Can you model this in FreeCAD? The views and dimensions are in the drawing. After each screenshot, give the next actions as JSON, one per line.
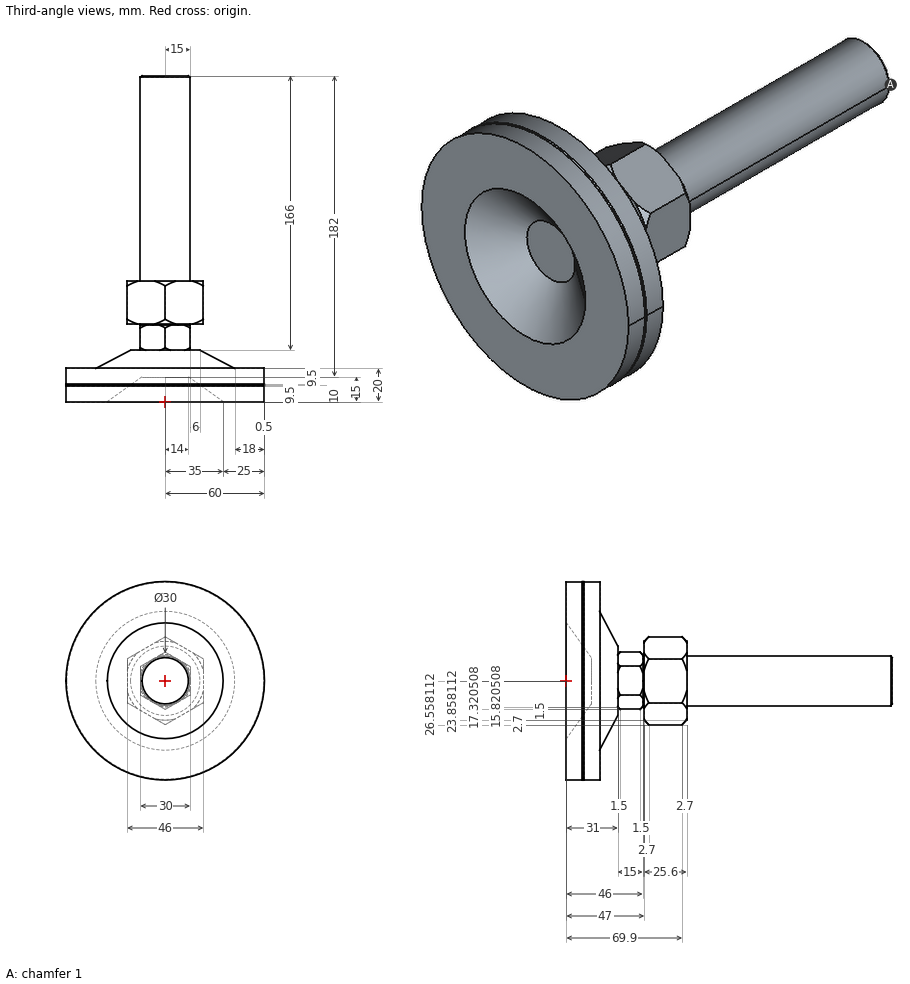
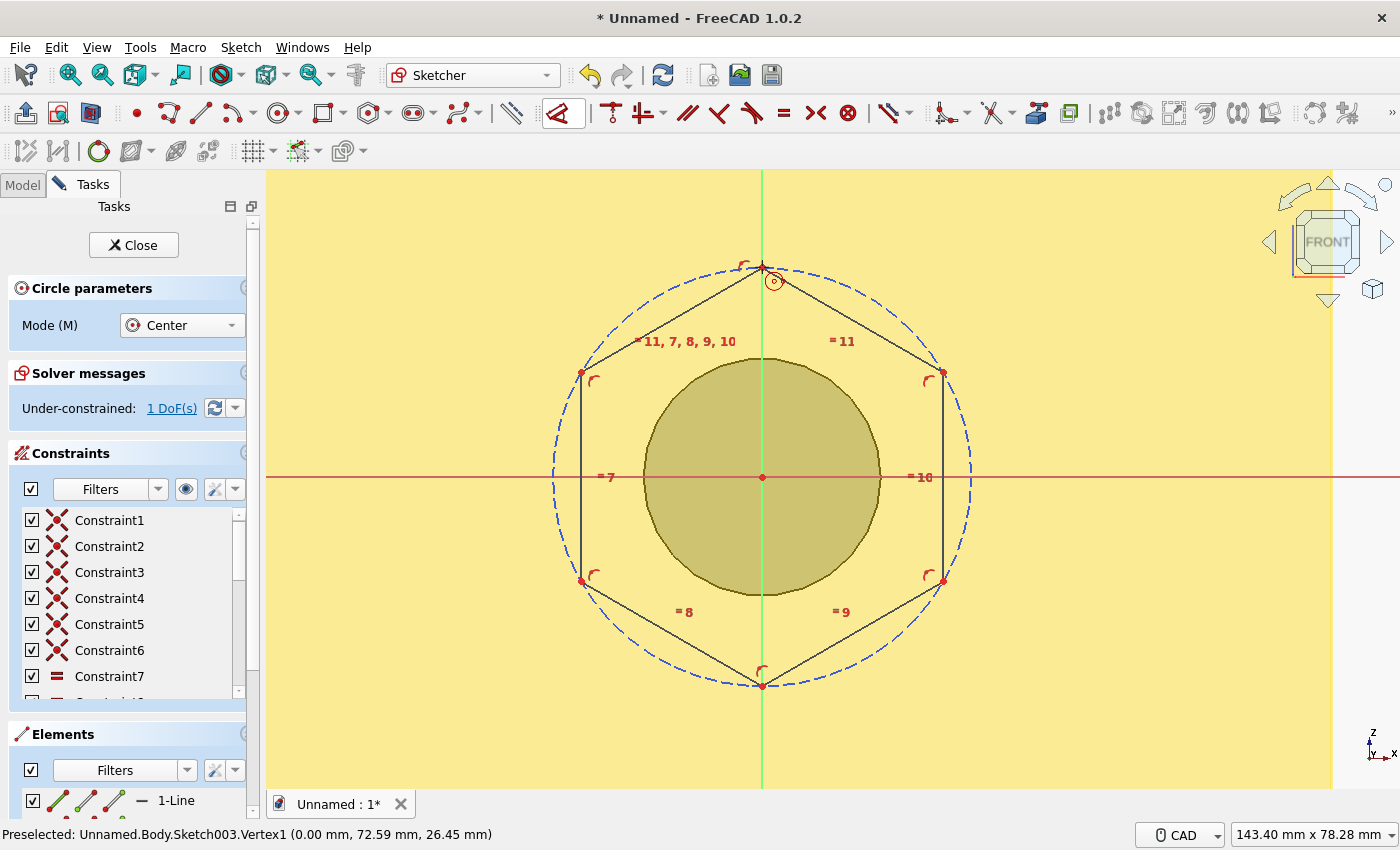
{"action": "left_click", "coordinate": [762, 477]}
{"action": "mouse_move", "coordinate": [846, 393]}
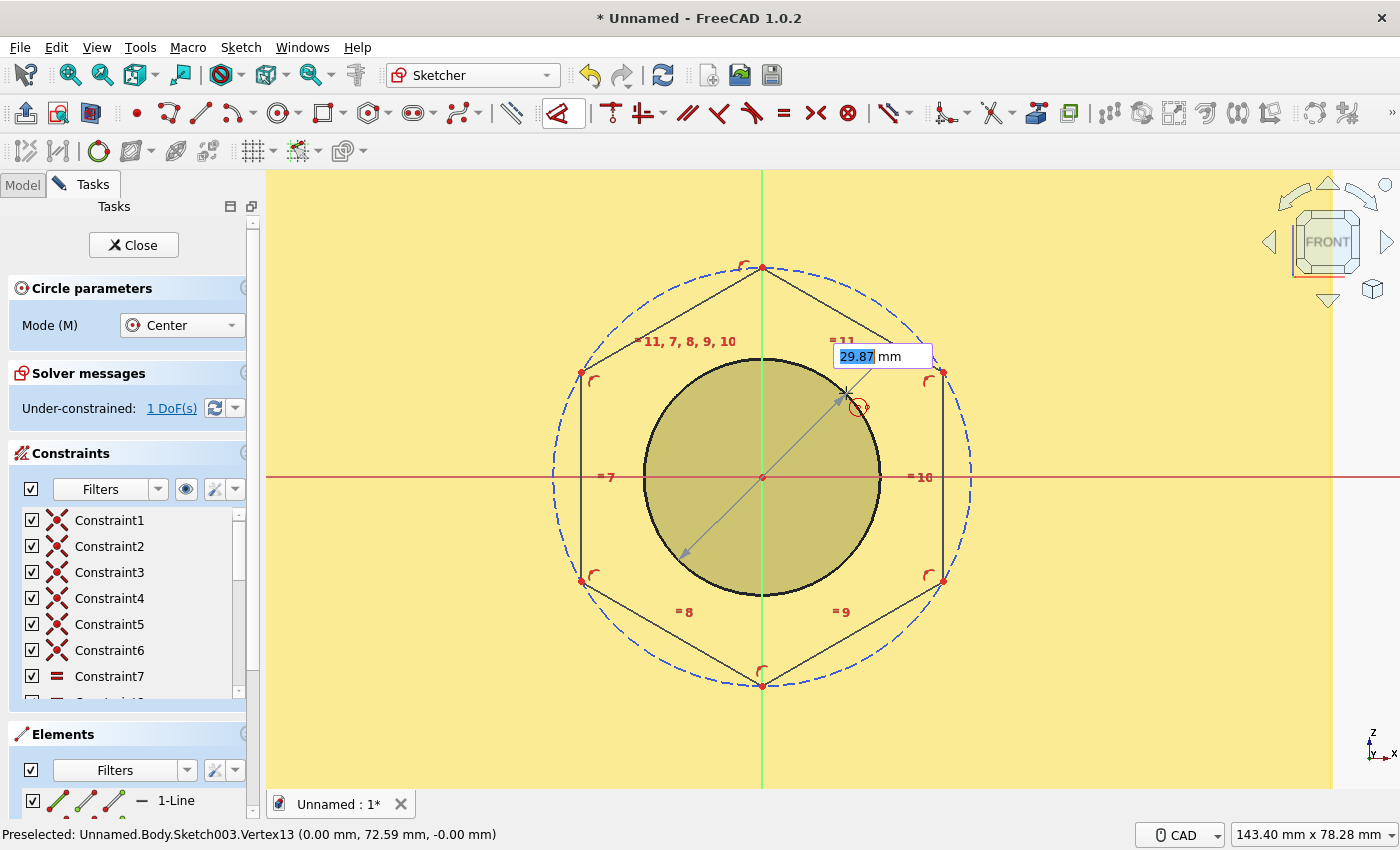
{"action": "type", "text": "30"}
{"action": "key", "text": "Return"}
{"action": "key", "text": "Escape"}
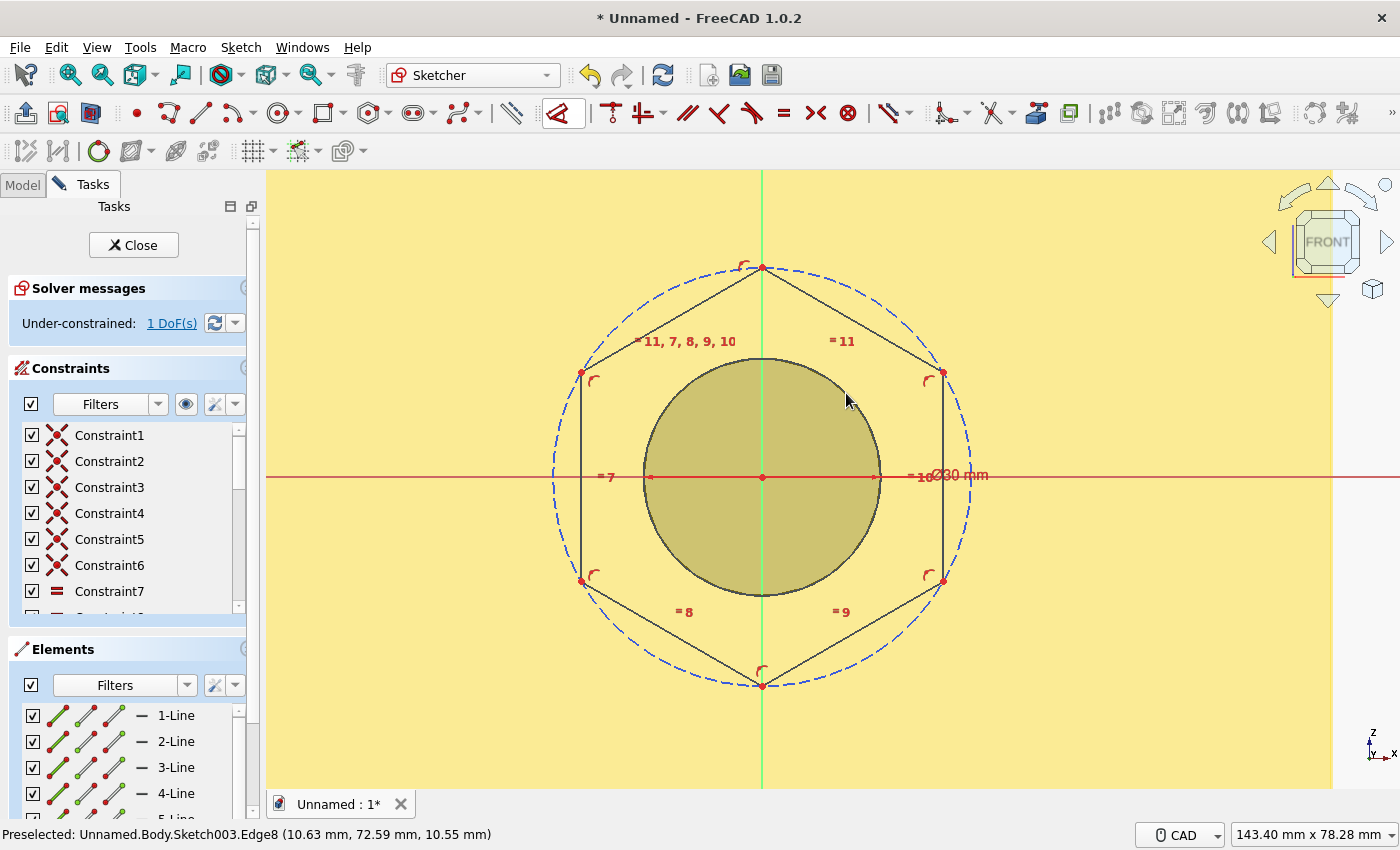
{"action": "left_click", "coordinate": [581, 373]}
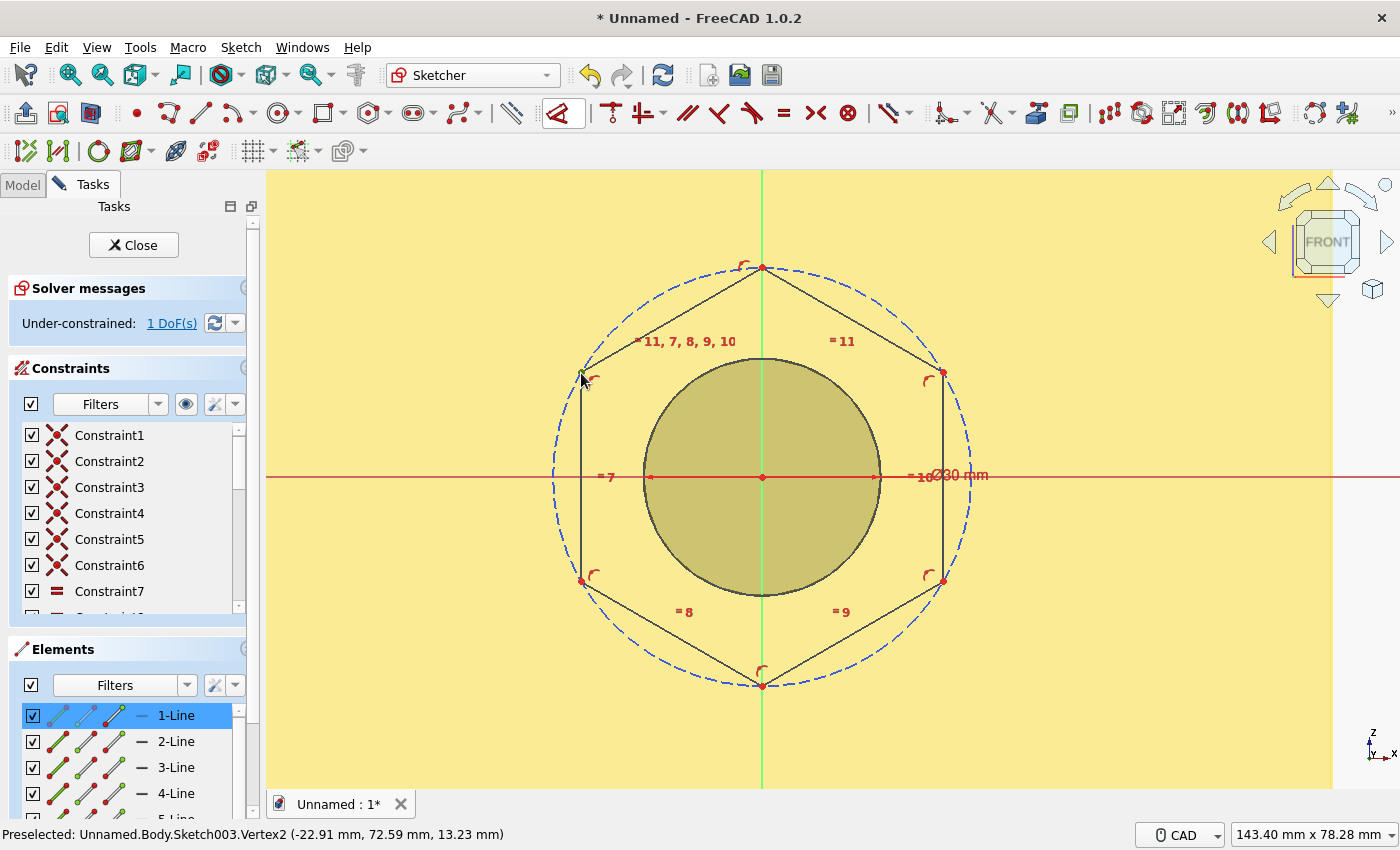
{"action": "left_click", "coordinate": [943, 582]}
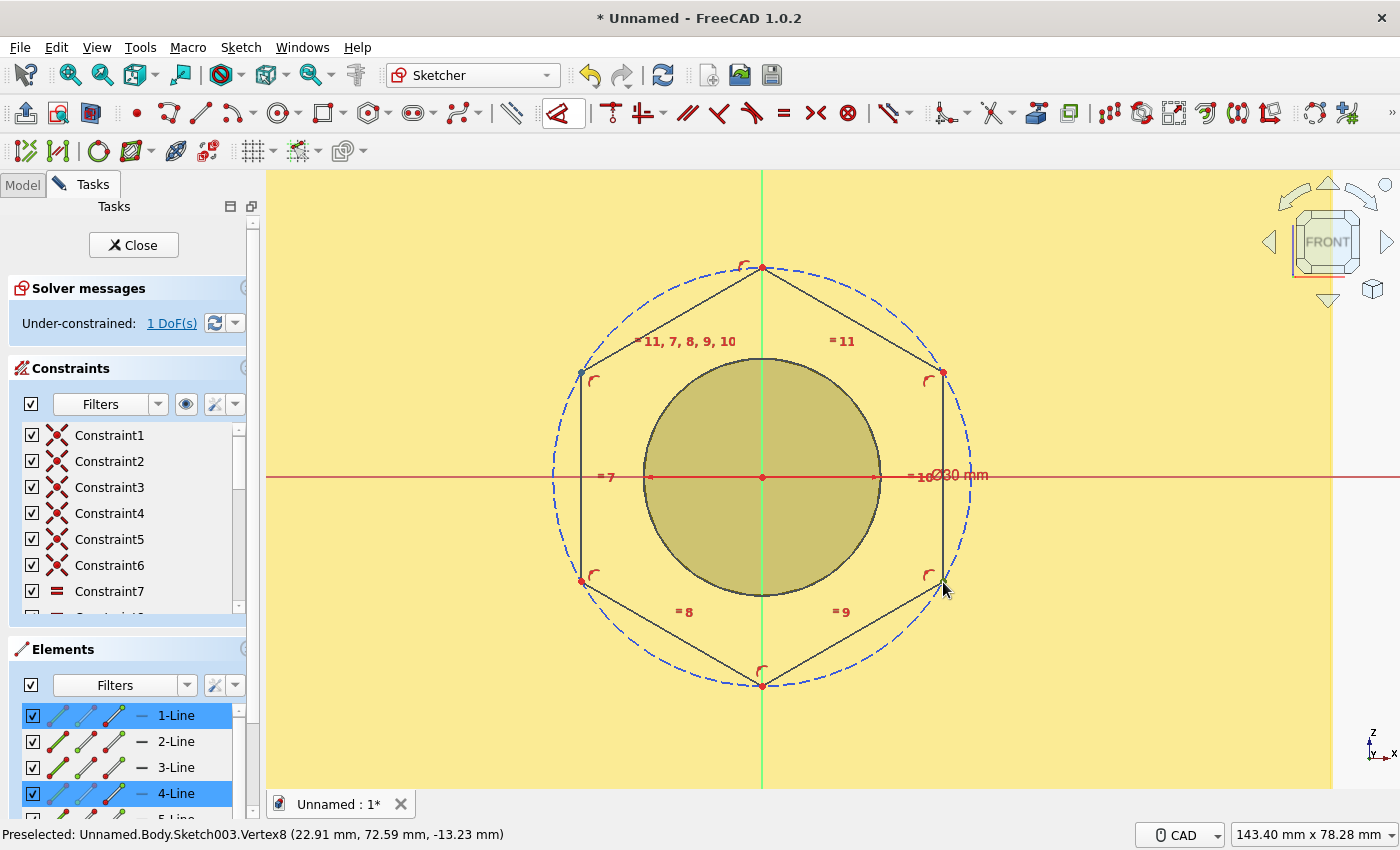
{"action": "key", "text": "l"}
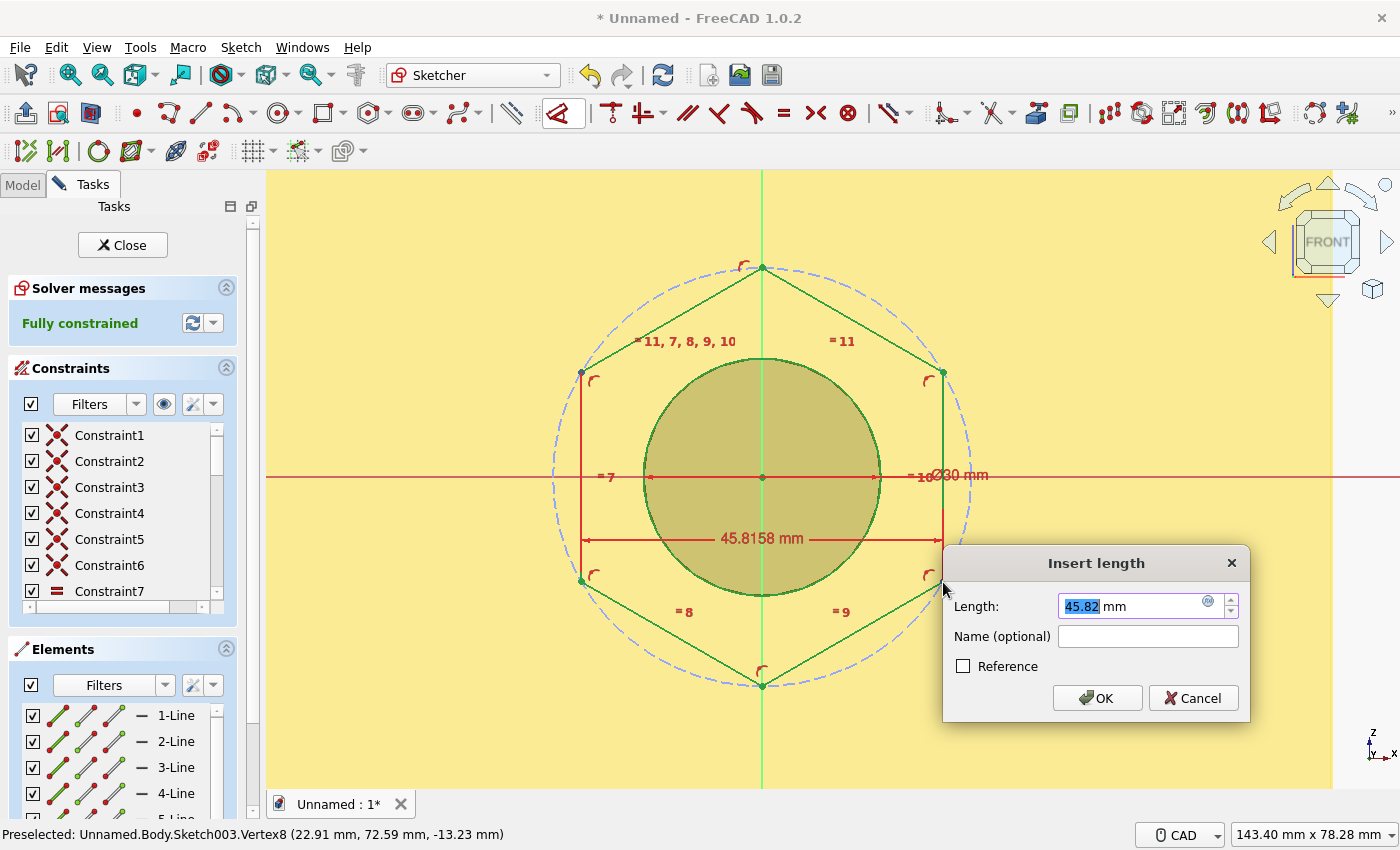
{"action": "type", "text": "46"}
{"action": "key", "text": "Return"}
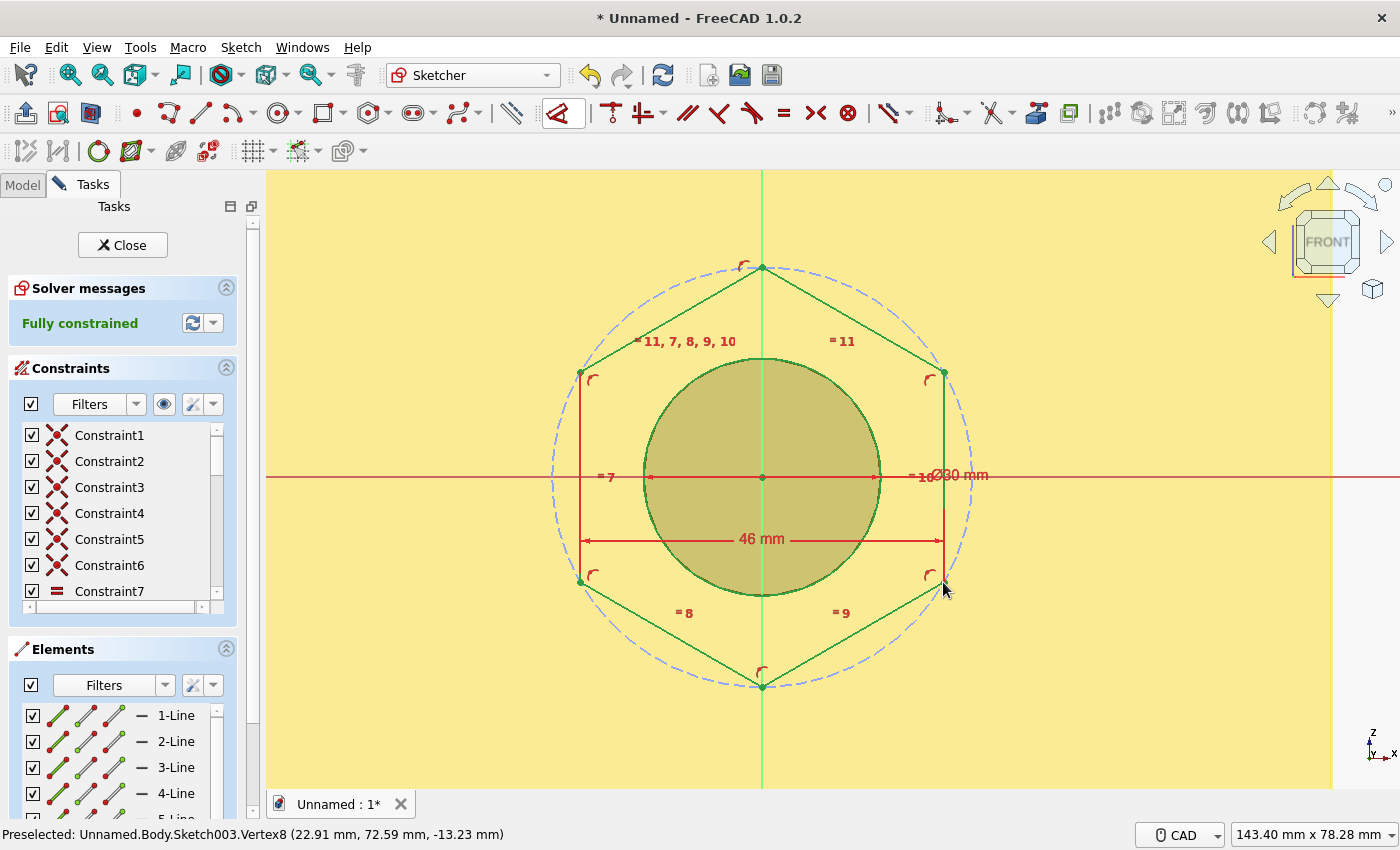
{"action": "left_click", "coordinate": [123, 245]}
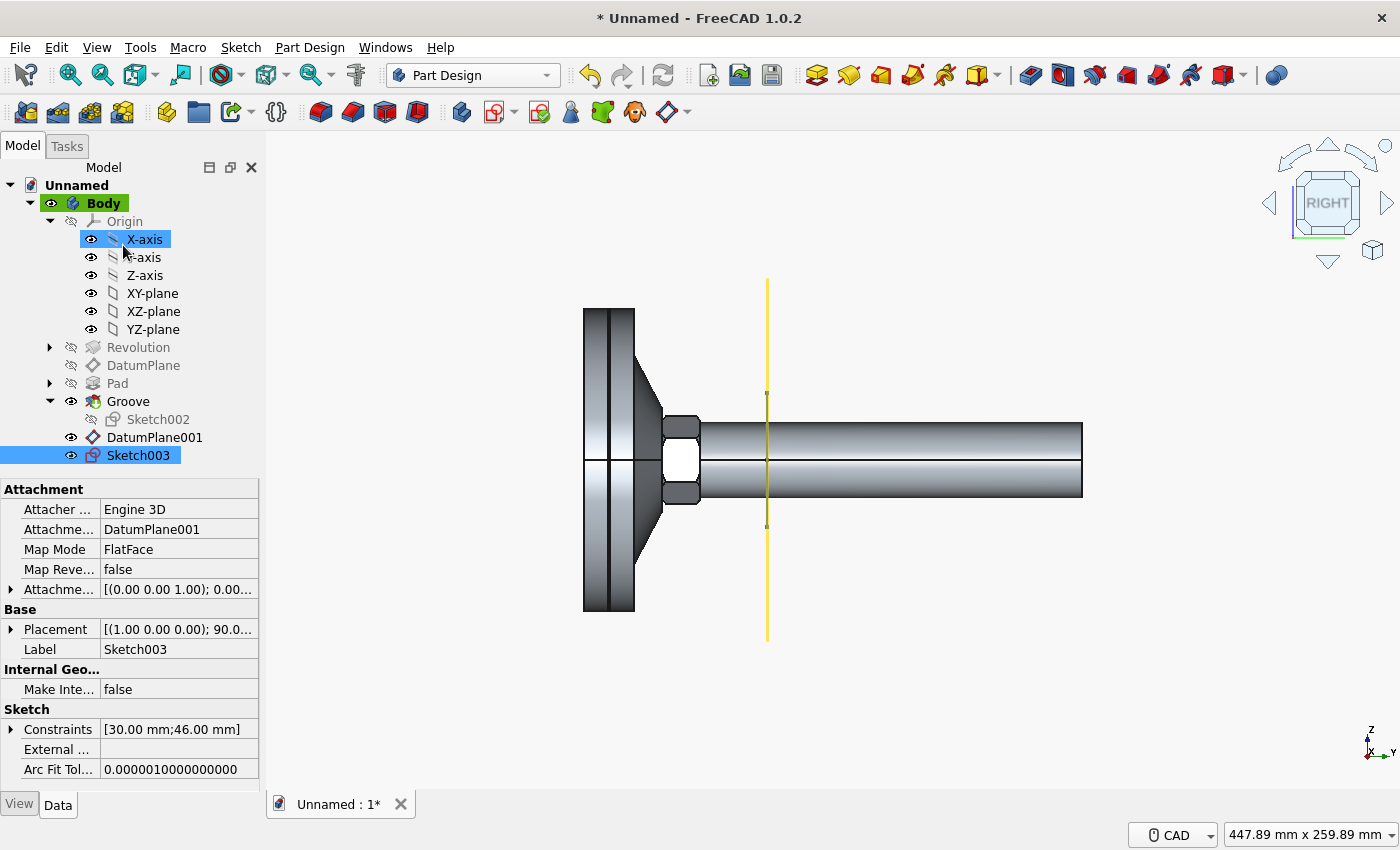
{"action": "left_click", "coordinate": [818, 76]}